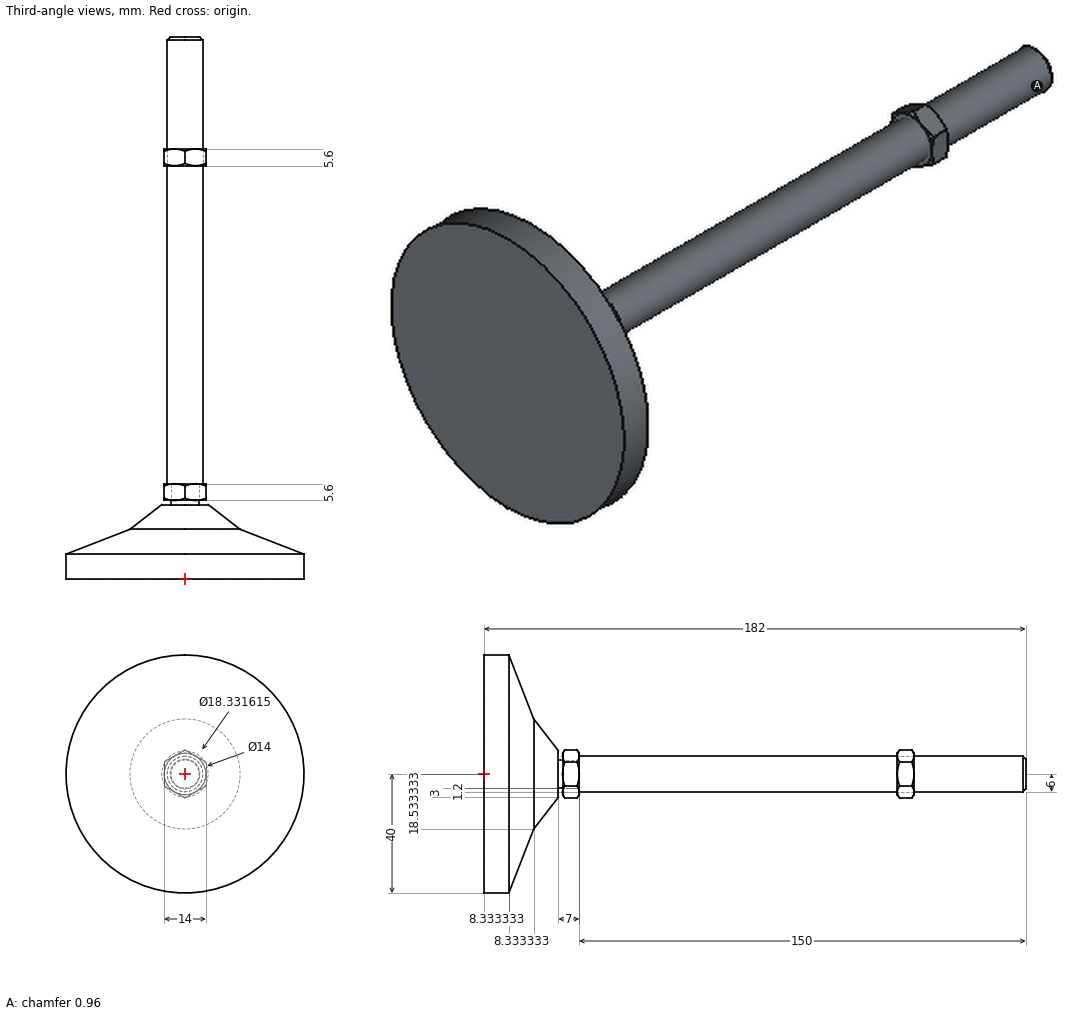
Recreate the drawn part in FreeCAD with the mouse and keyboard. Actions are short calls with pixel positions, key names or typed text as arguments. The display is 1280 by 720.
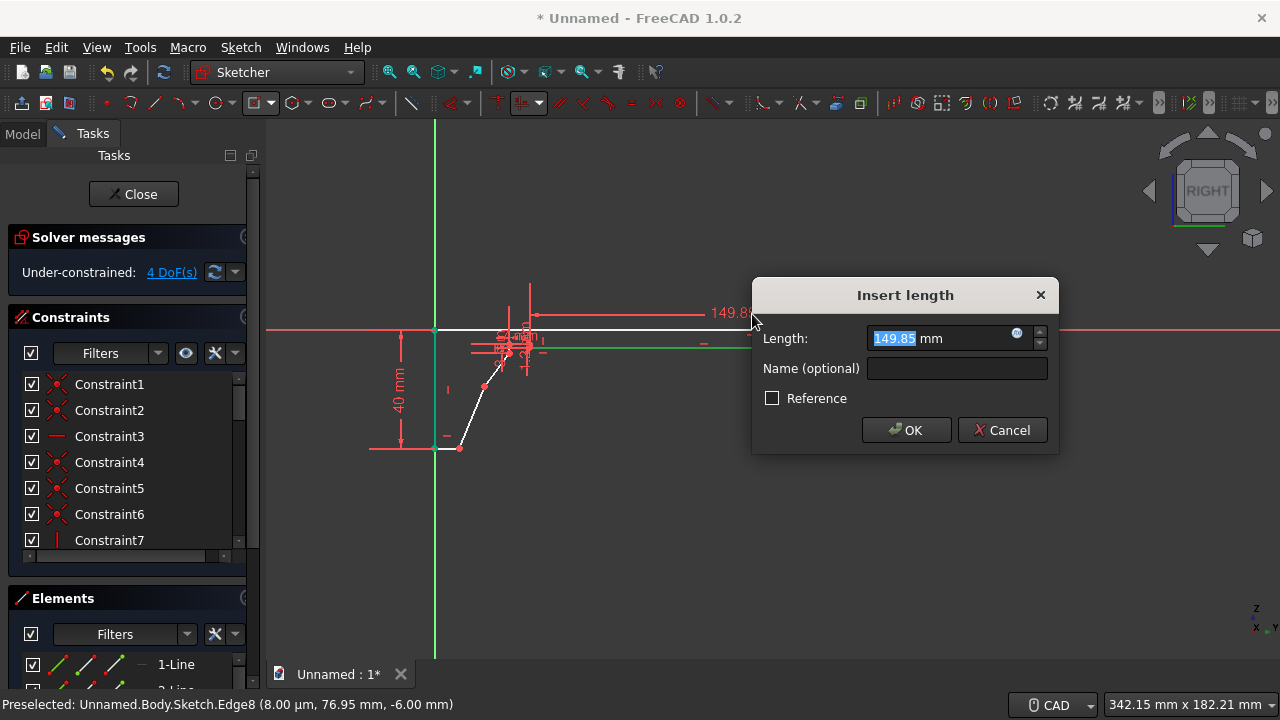
text(150)
key(Return)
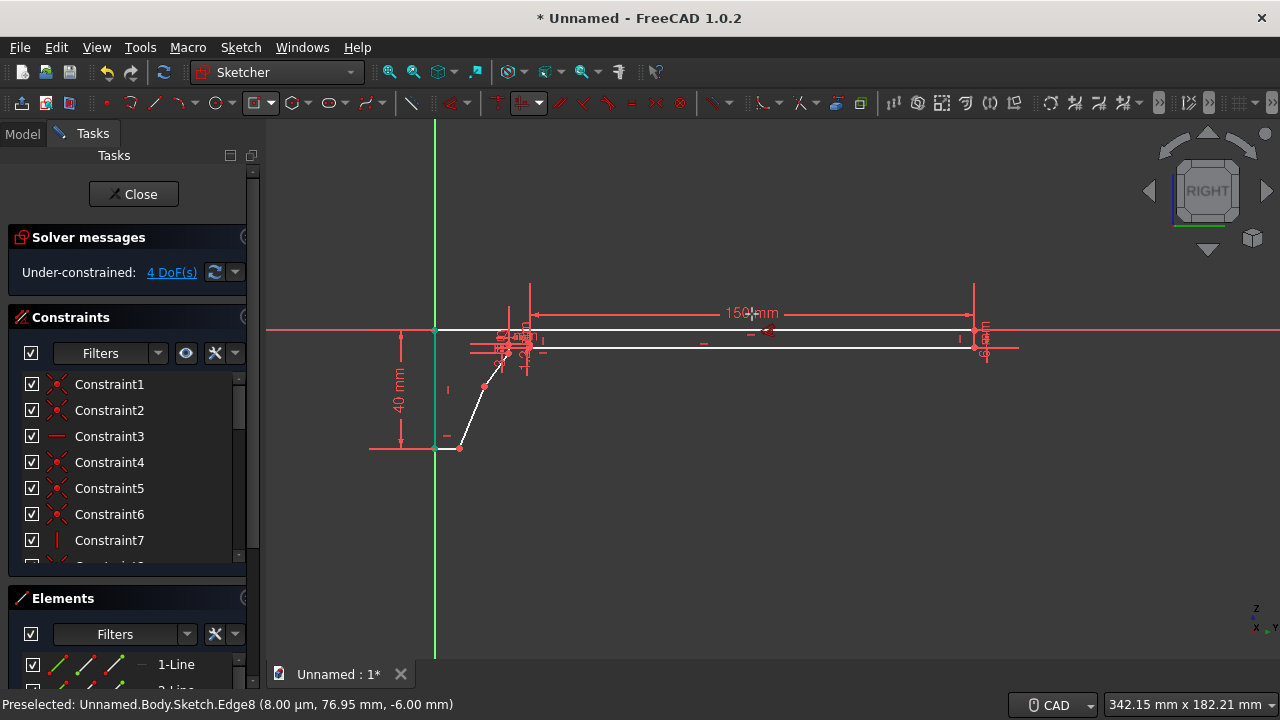
click(812, 330)
click(581, 296)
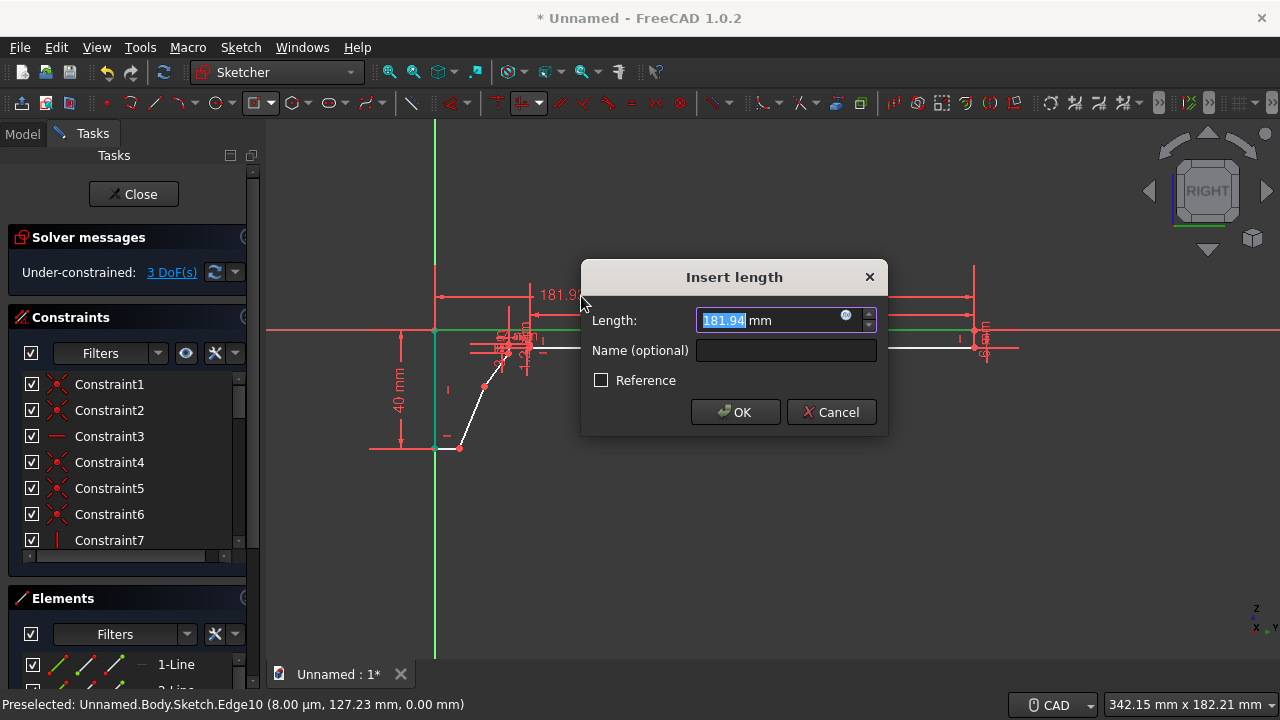
text(182)
key(Return)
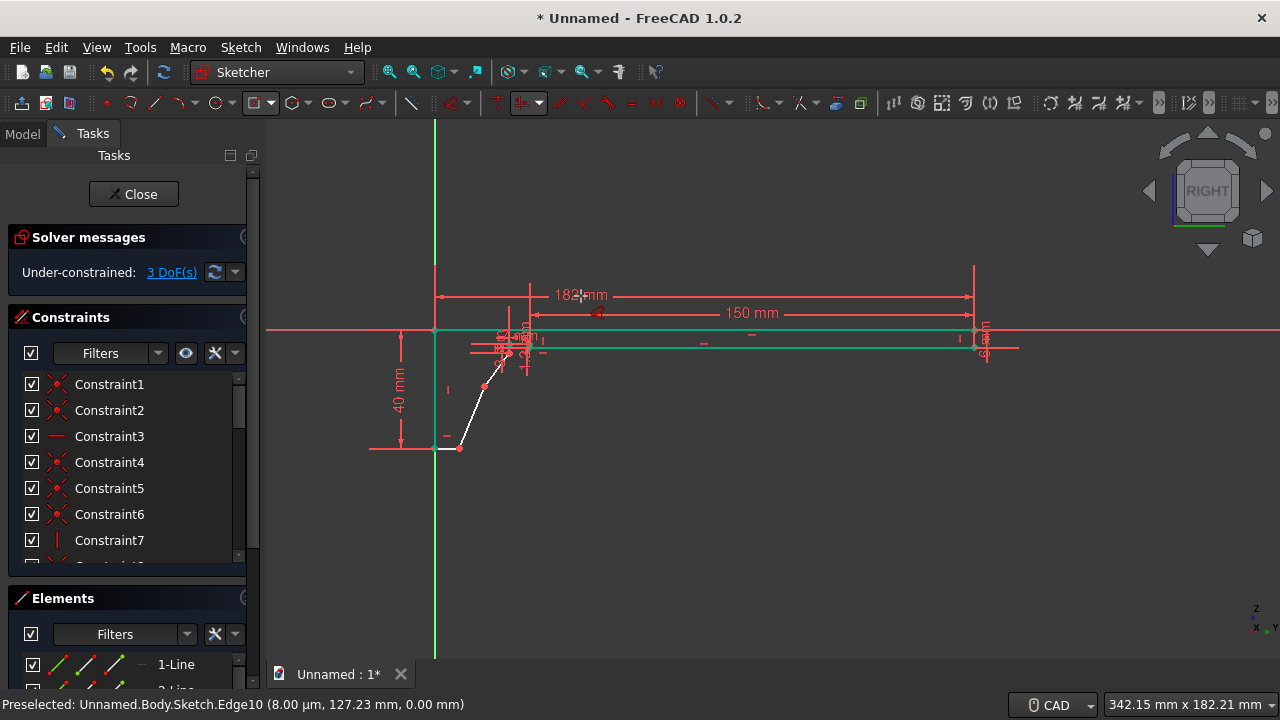
scroll(445, 449, up, 3)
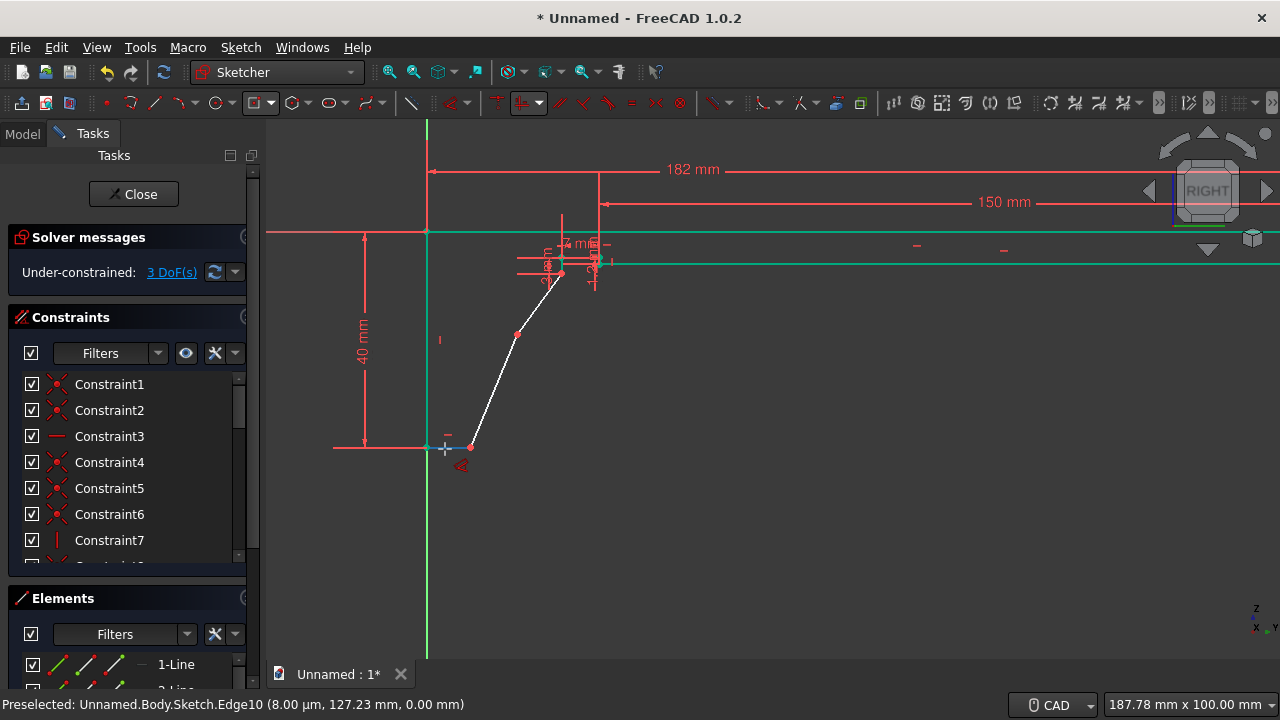
click(444, 448)
click(449, 482)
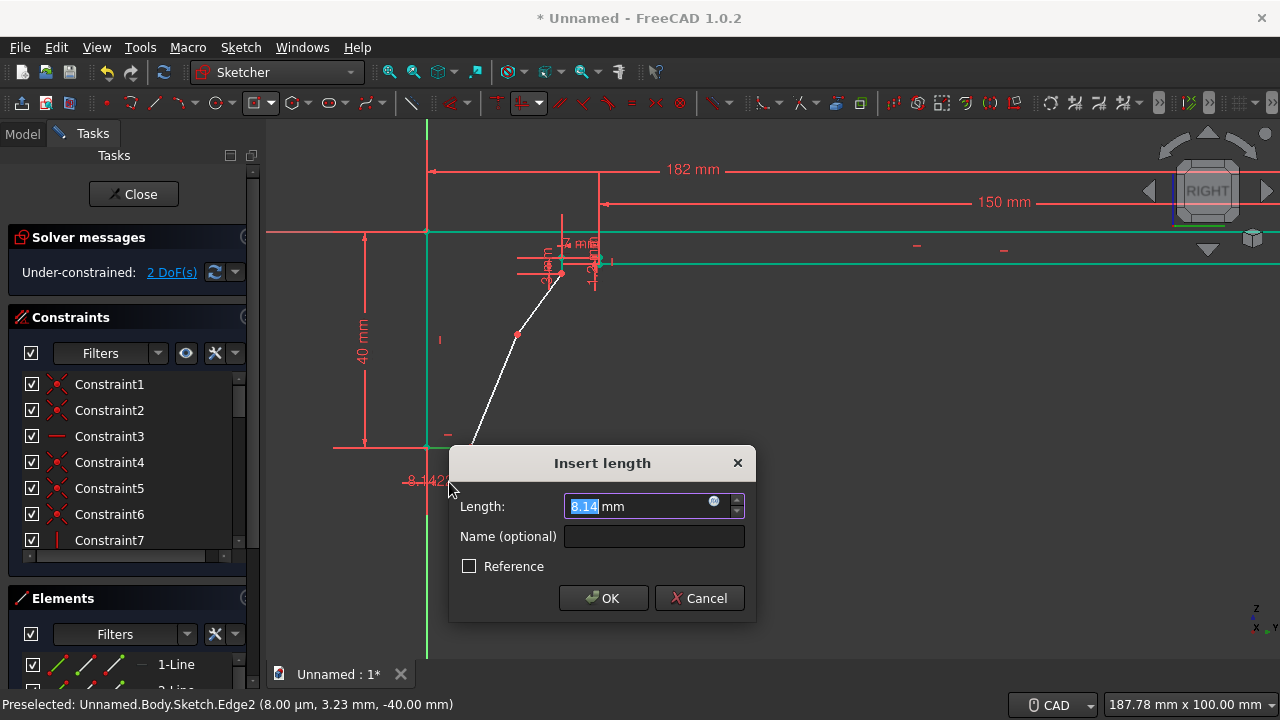
text(8.333333)
key(Return)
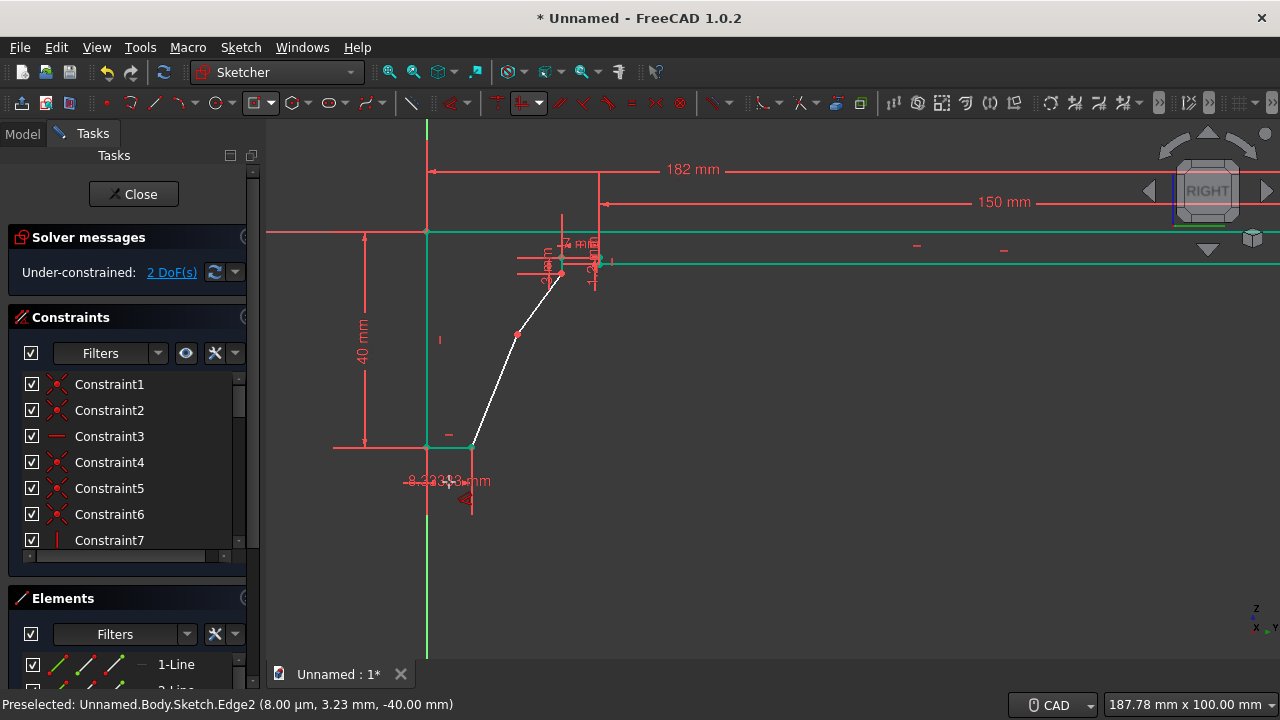
click(485, 414)
click(494, 301)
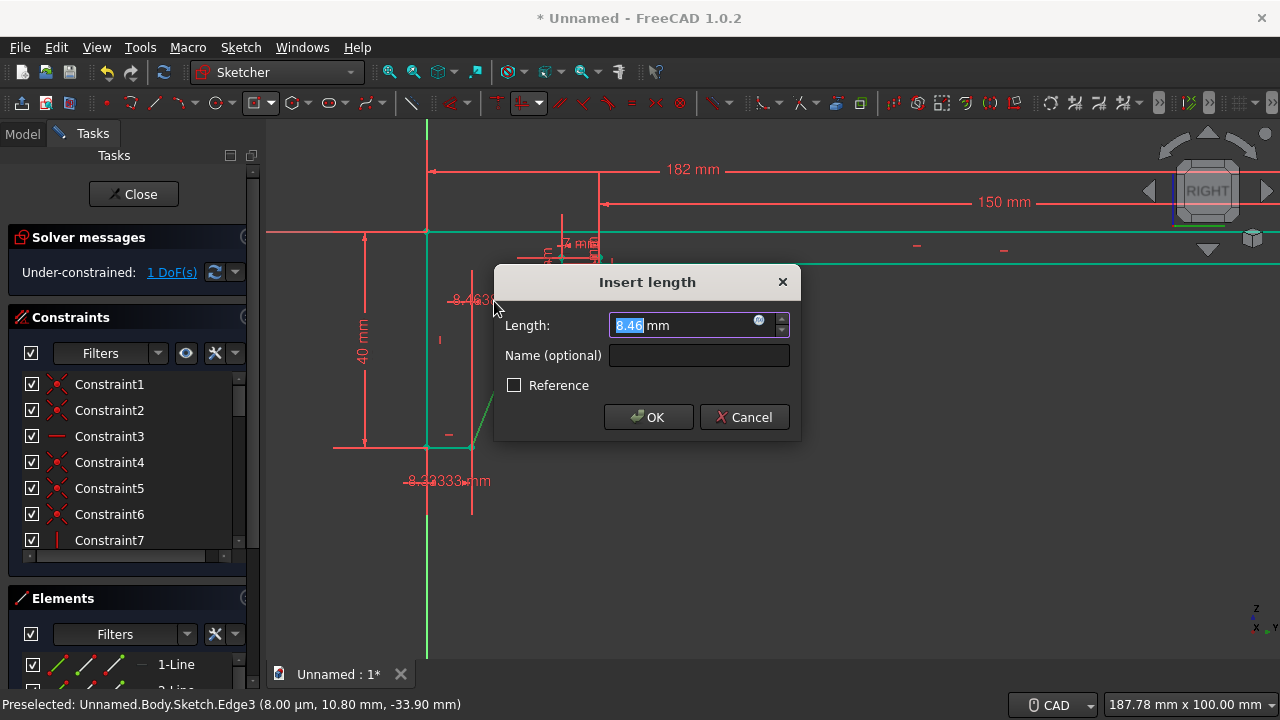
text(8.333333)
key(Return)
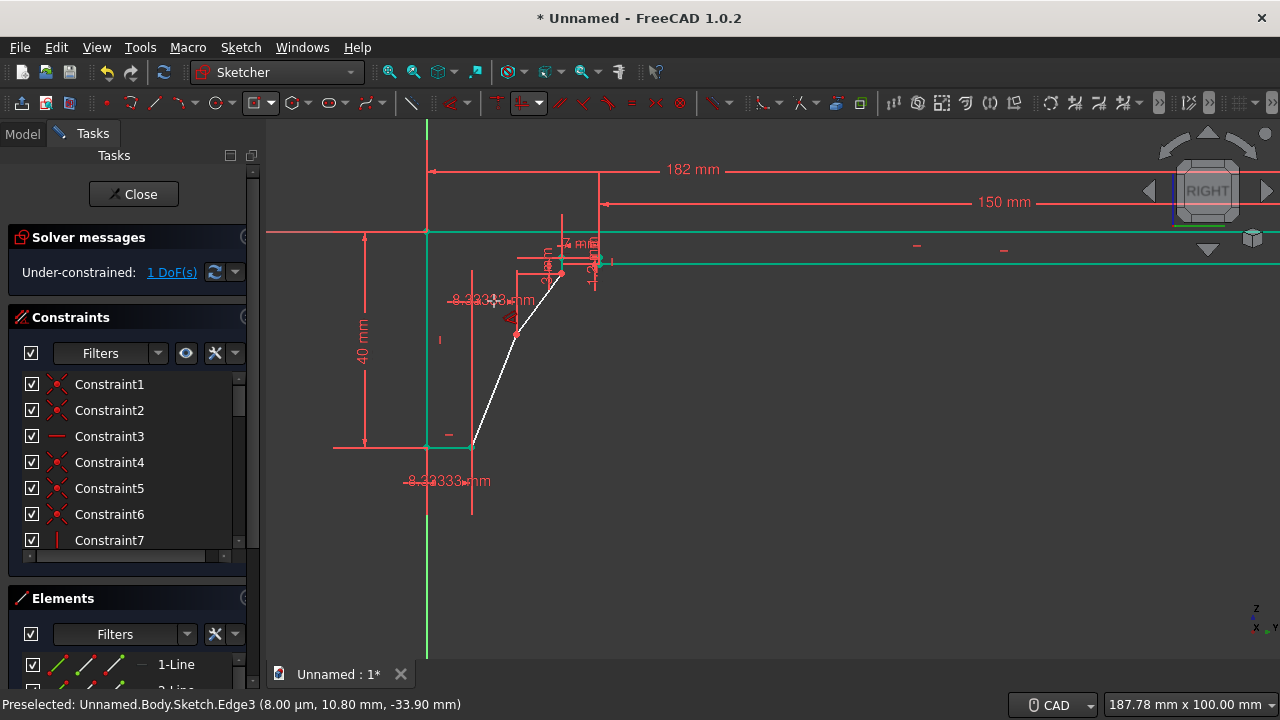
click(517, 335)
click(393, 283)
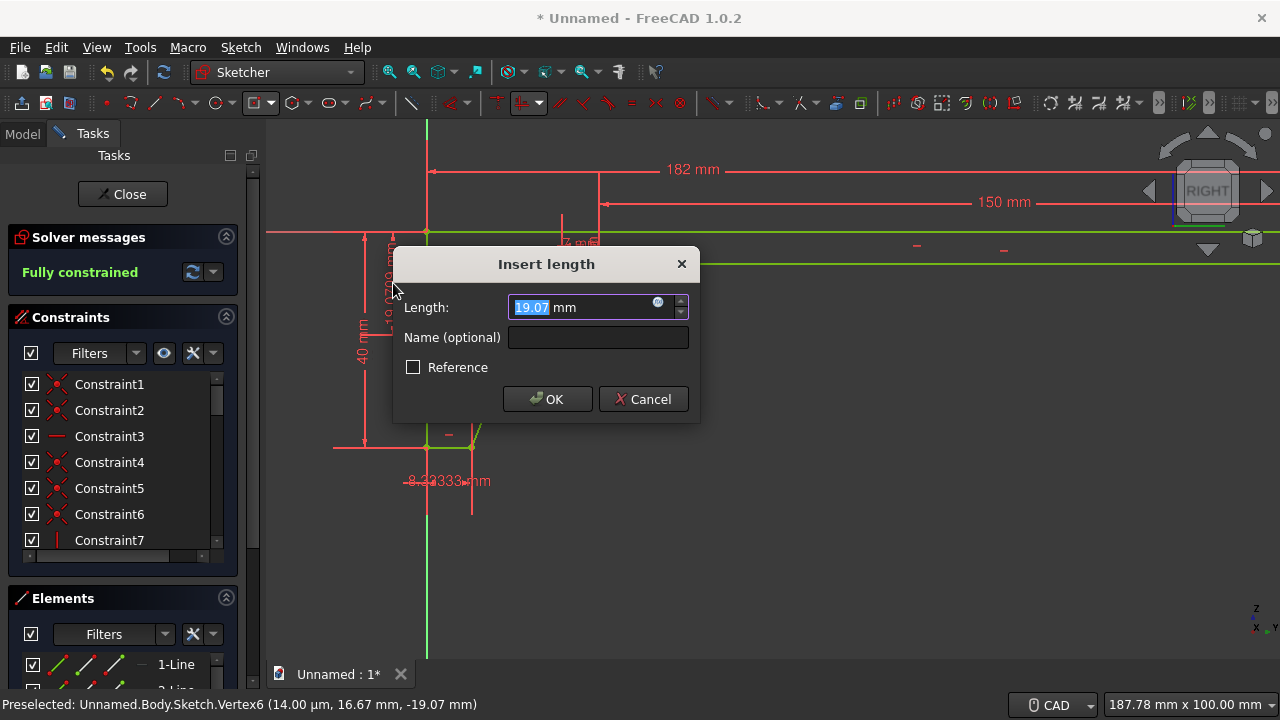
text(18.533333)
key(Return)
key(Escape)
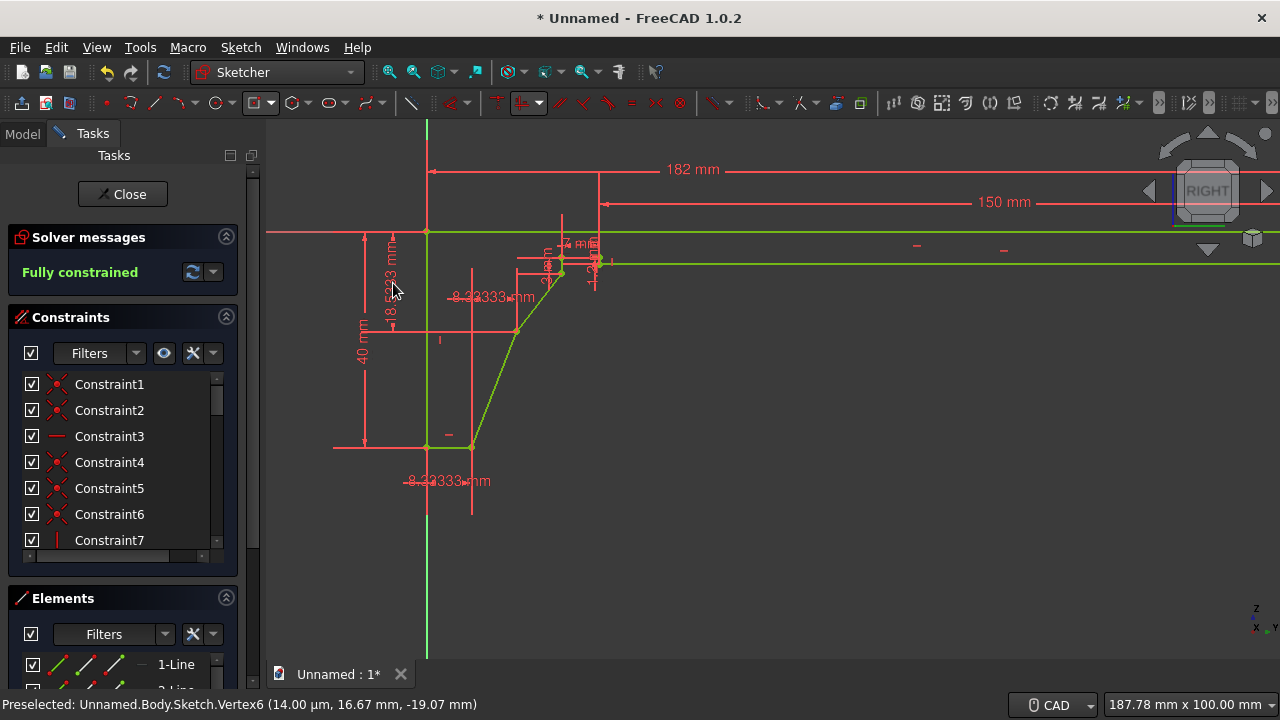
click(123, 194)